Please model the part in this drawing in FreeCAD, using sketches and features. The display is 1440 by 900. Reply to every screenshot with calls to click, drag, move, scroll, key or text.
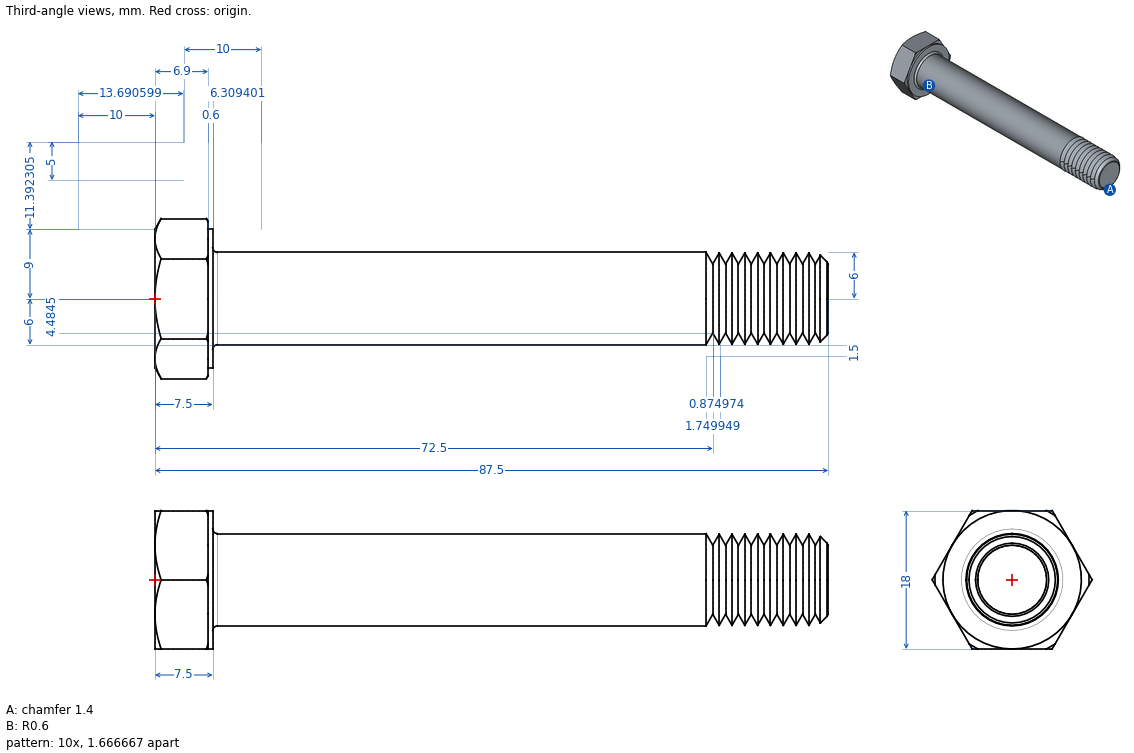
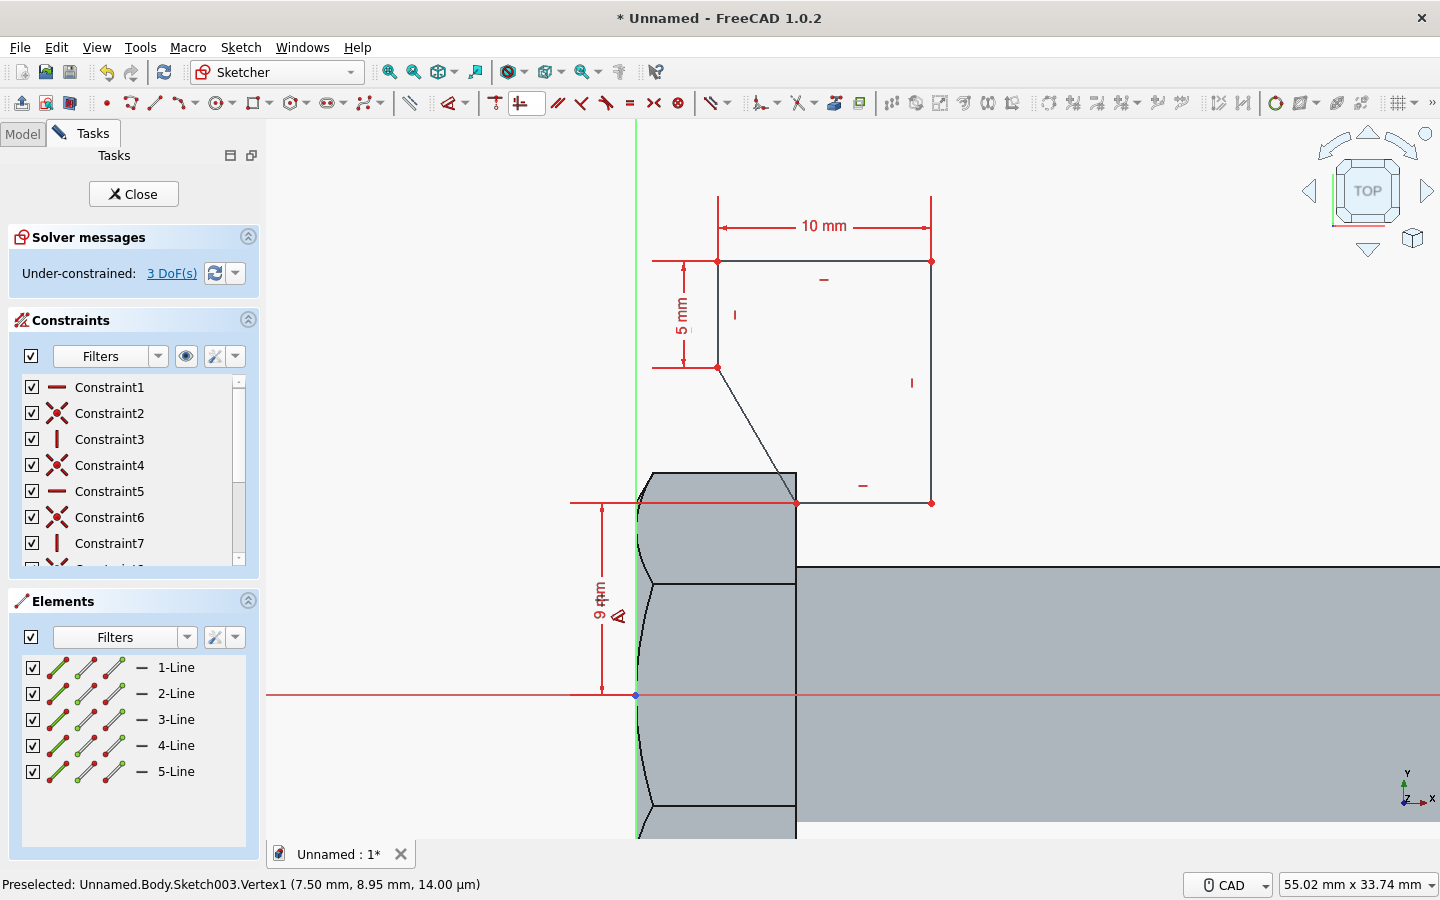
click(796, 503)
click(716, 729)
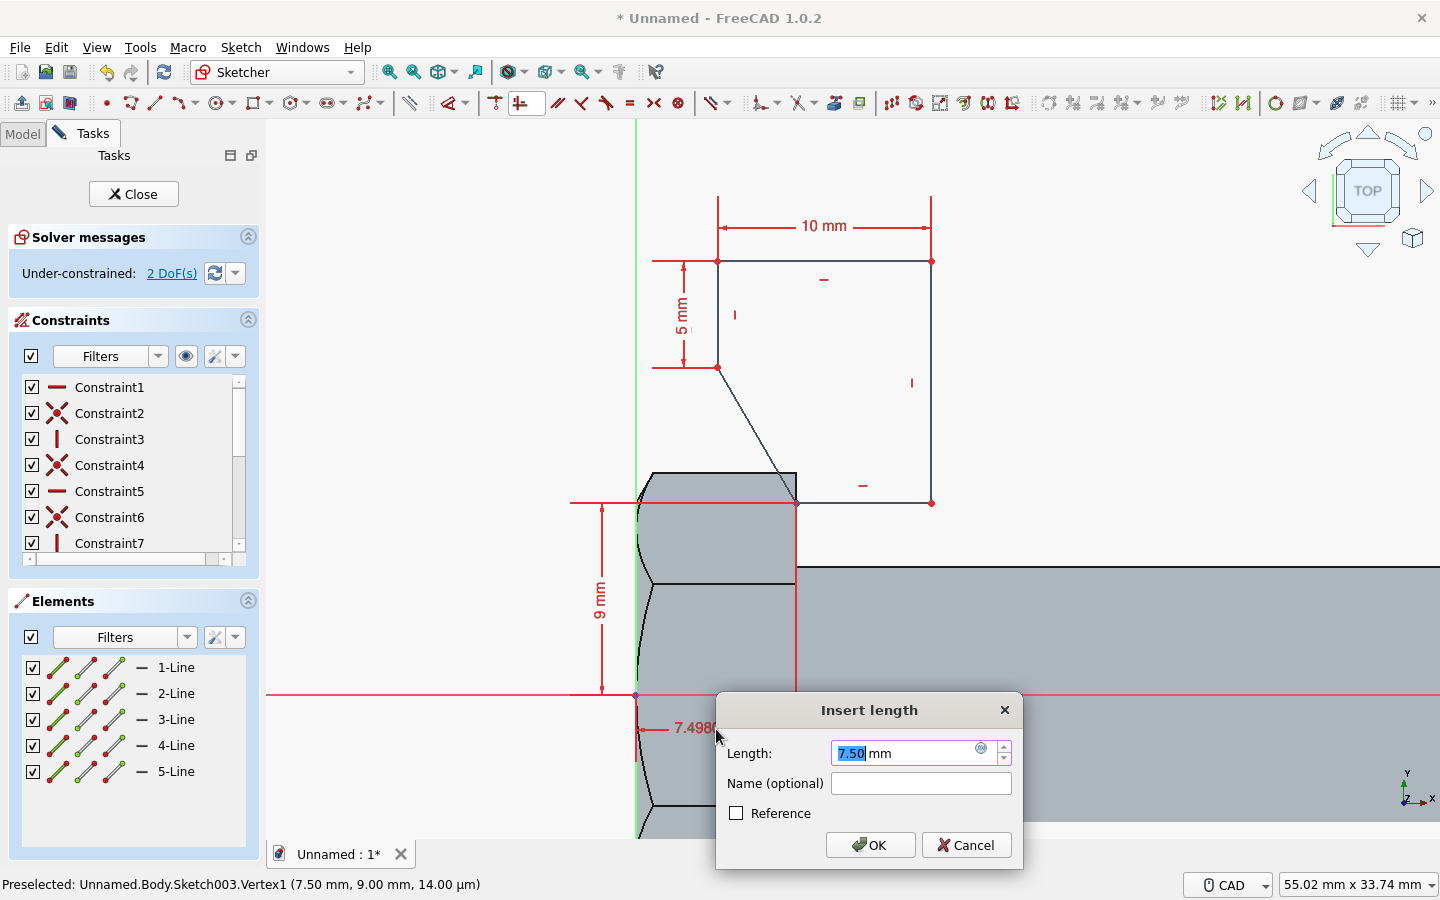
text(7.5)
key(Return)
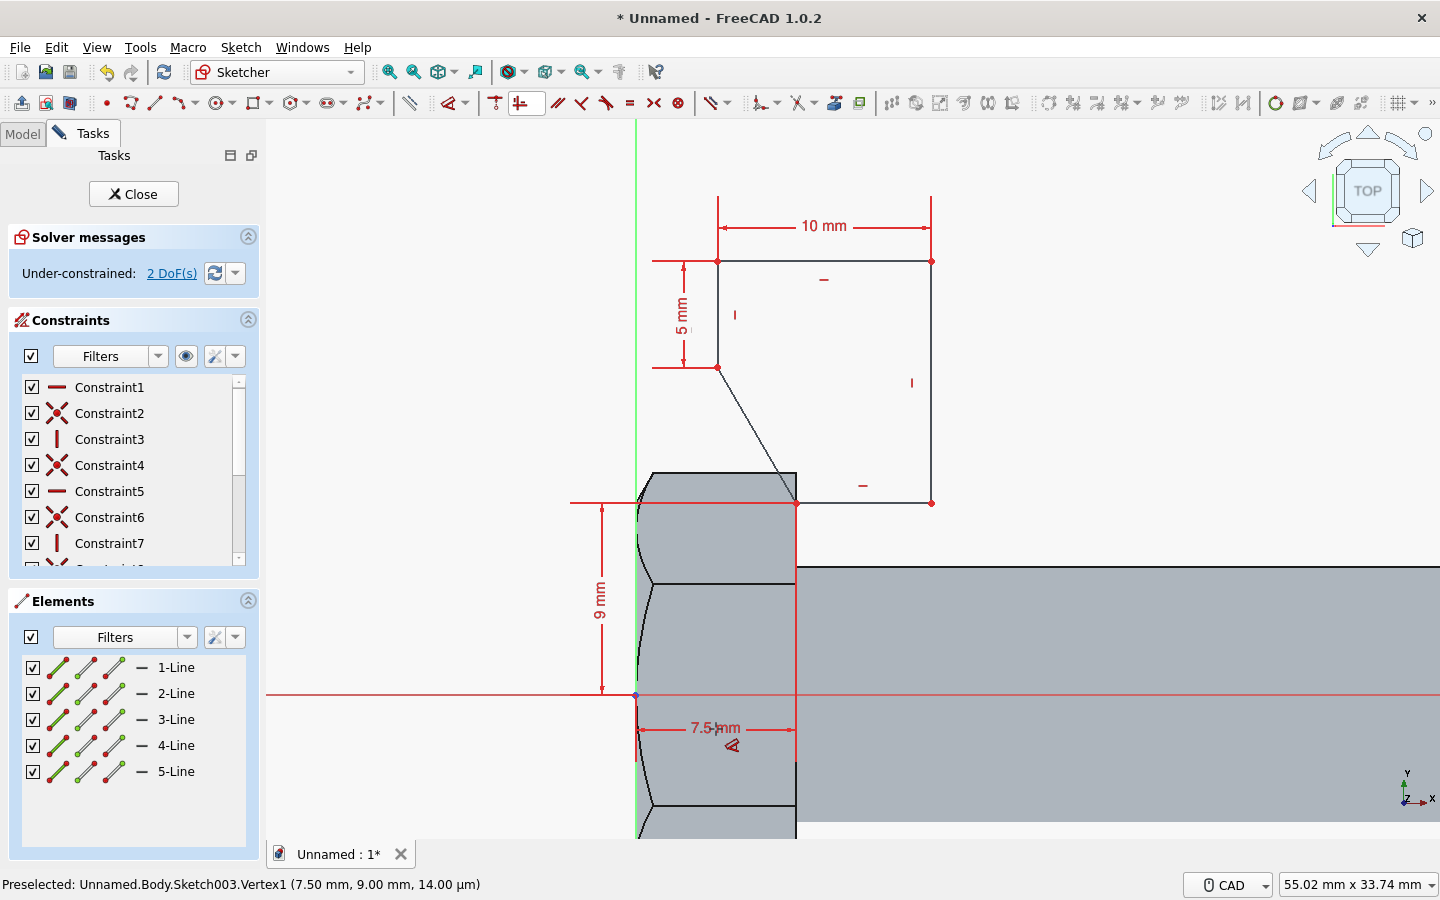
click(837, 503)
click(864, 537)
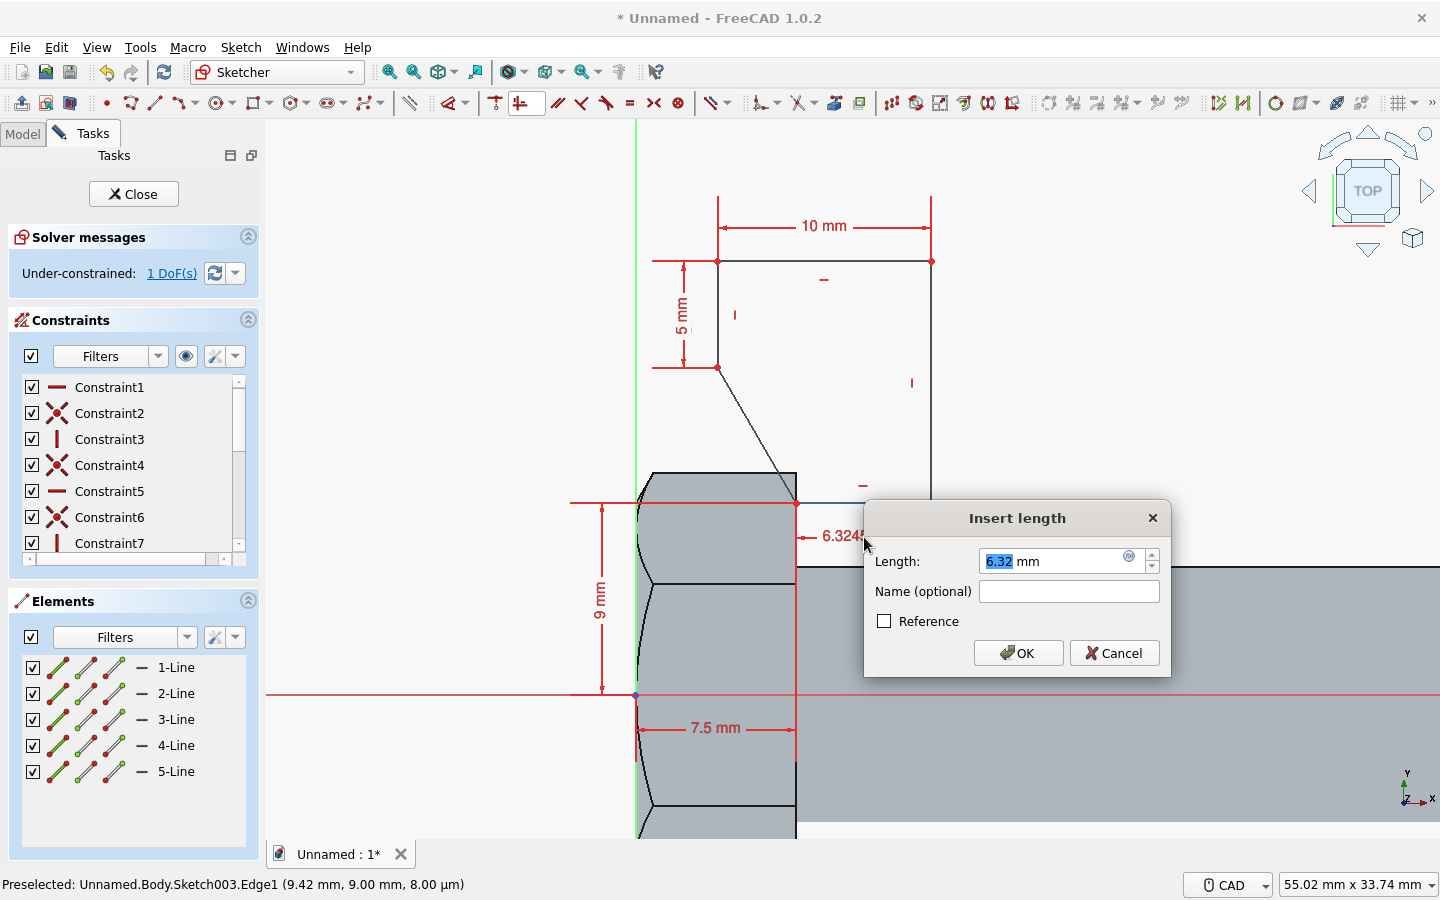
text(6.309401)
key(Return)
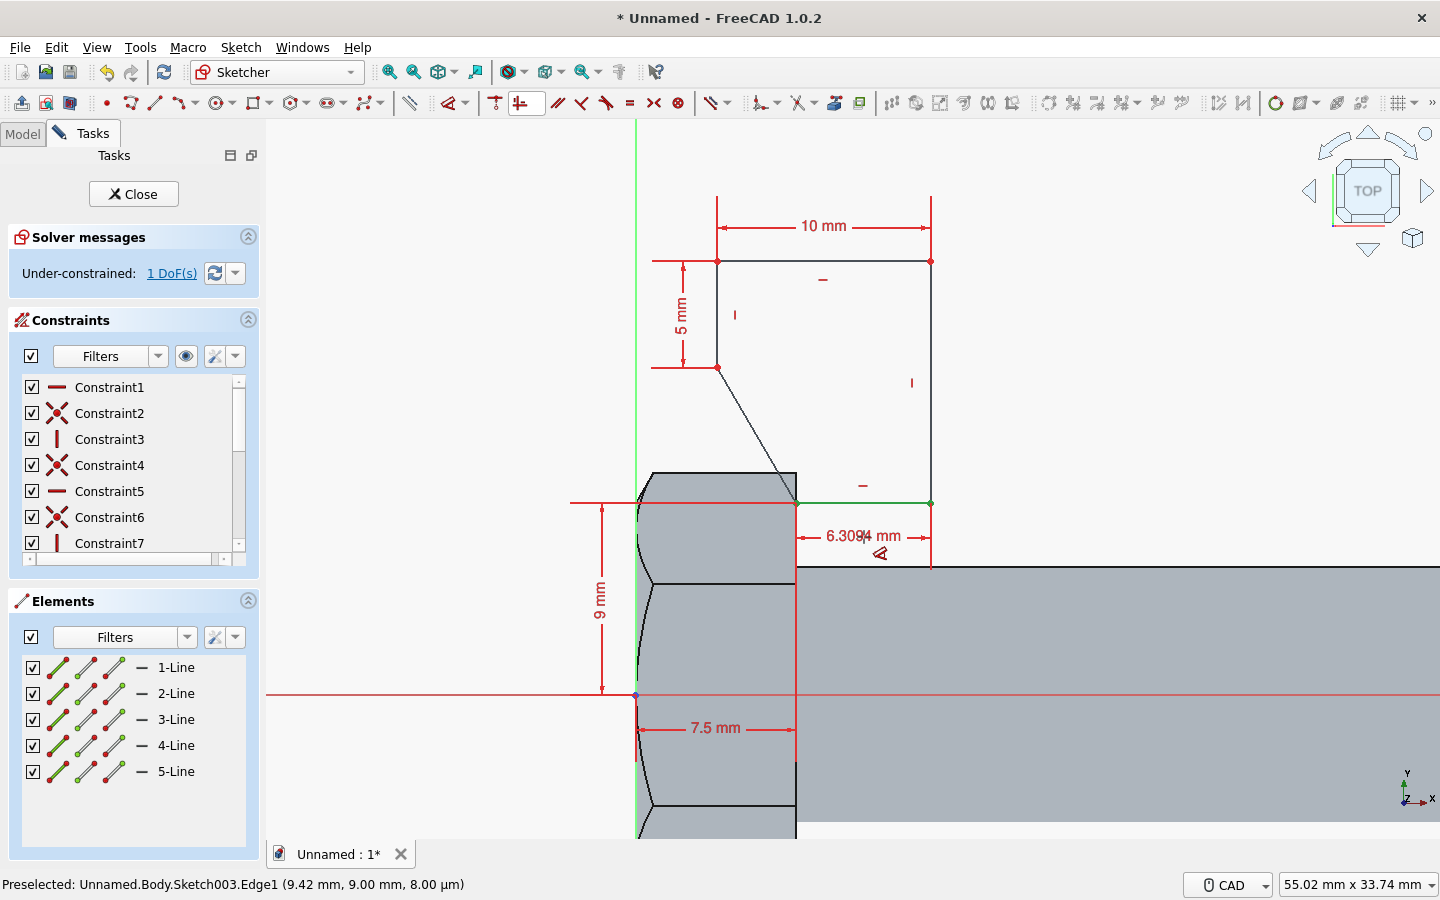
click(931, 430)
click(965, 382)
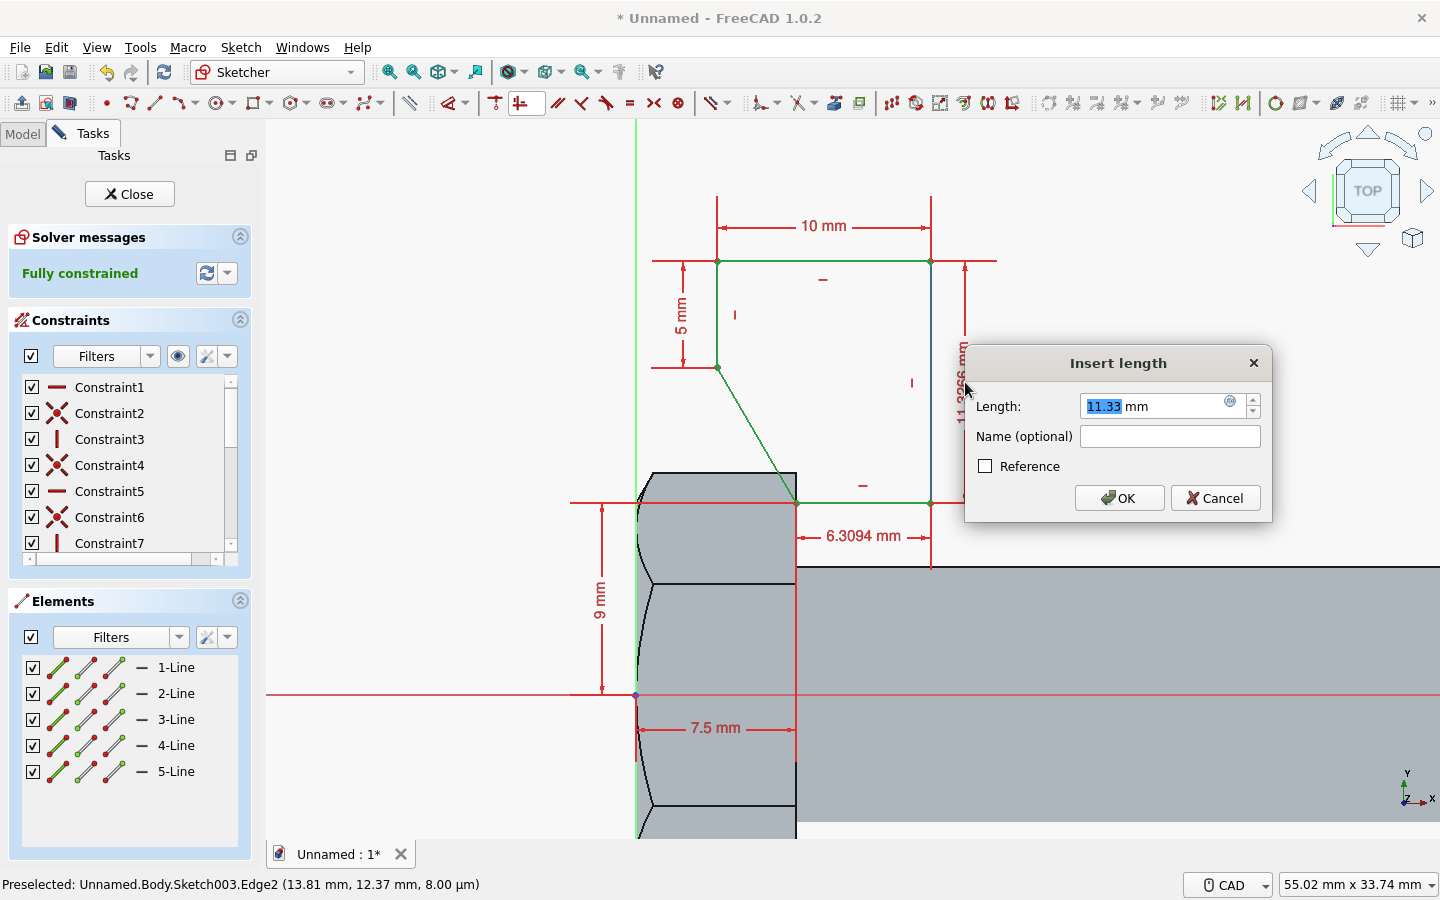
text(11.392305)
key(Return)
key(Escape)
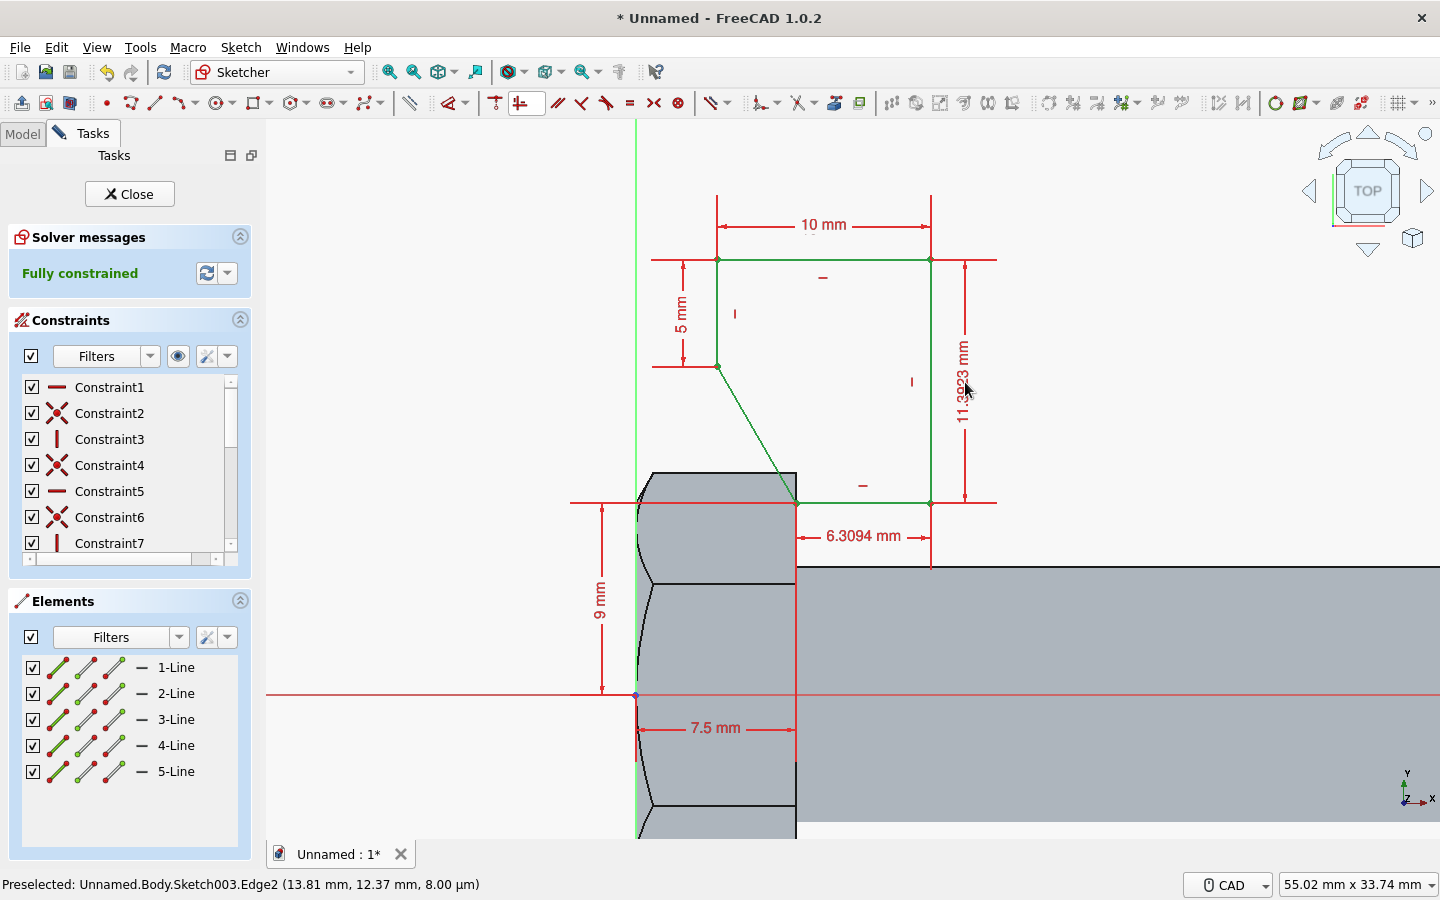
click(130, 194)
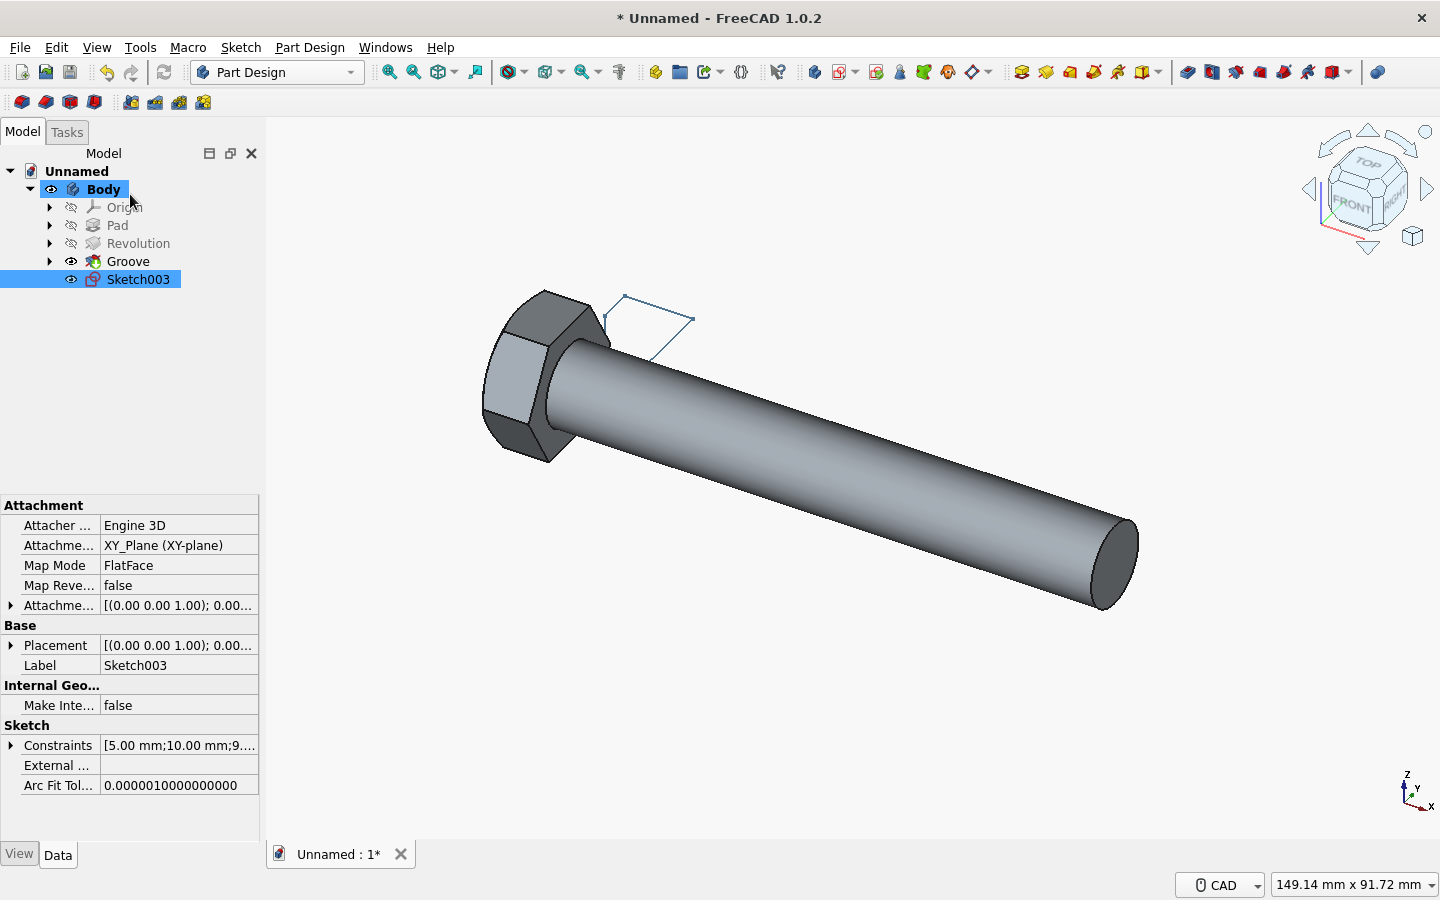
click(1236, 72)